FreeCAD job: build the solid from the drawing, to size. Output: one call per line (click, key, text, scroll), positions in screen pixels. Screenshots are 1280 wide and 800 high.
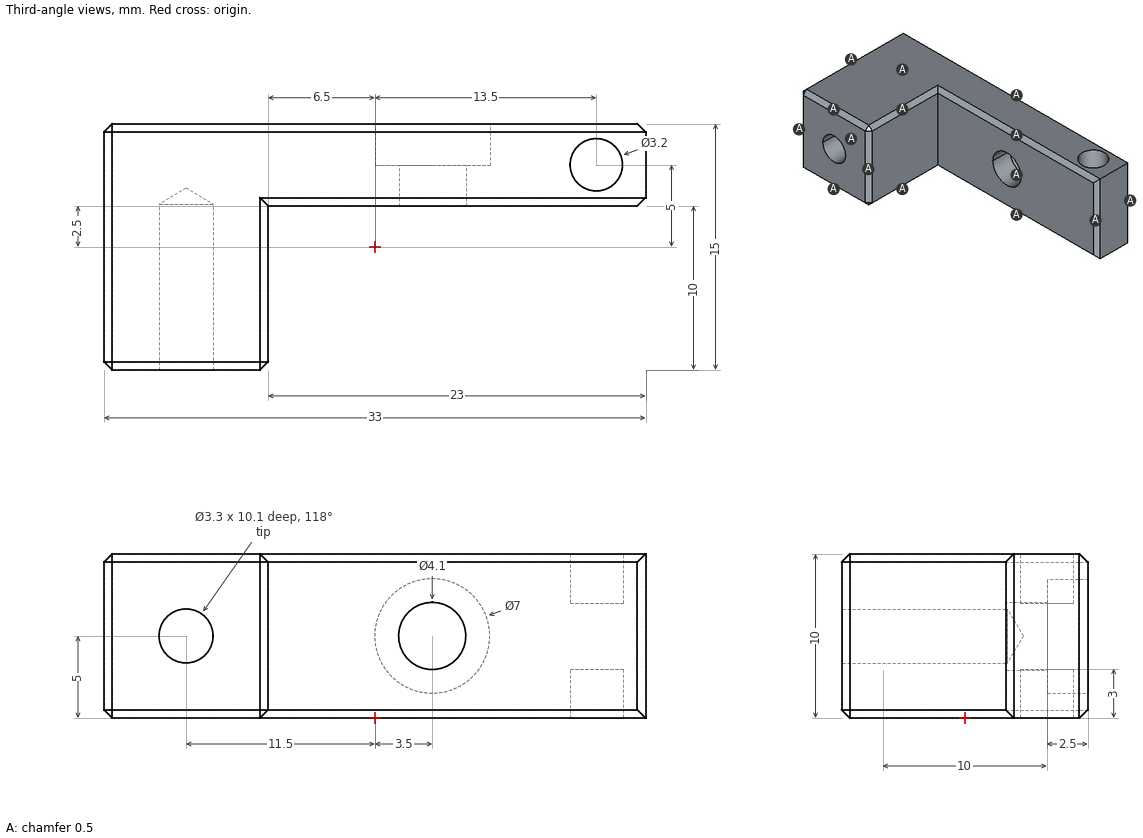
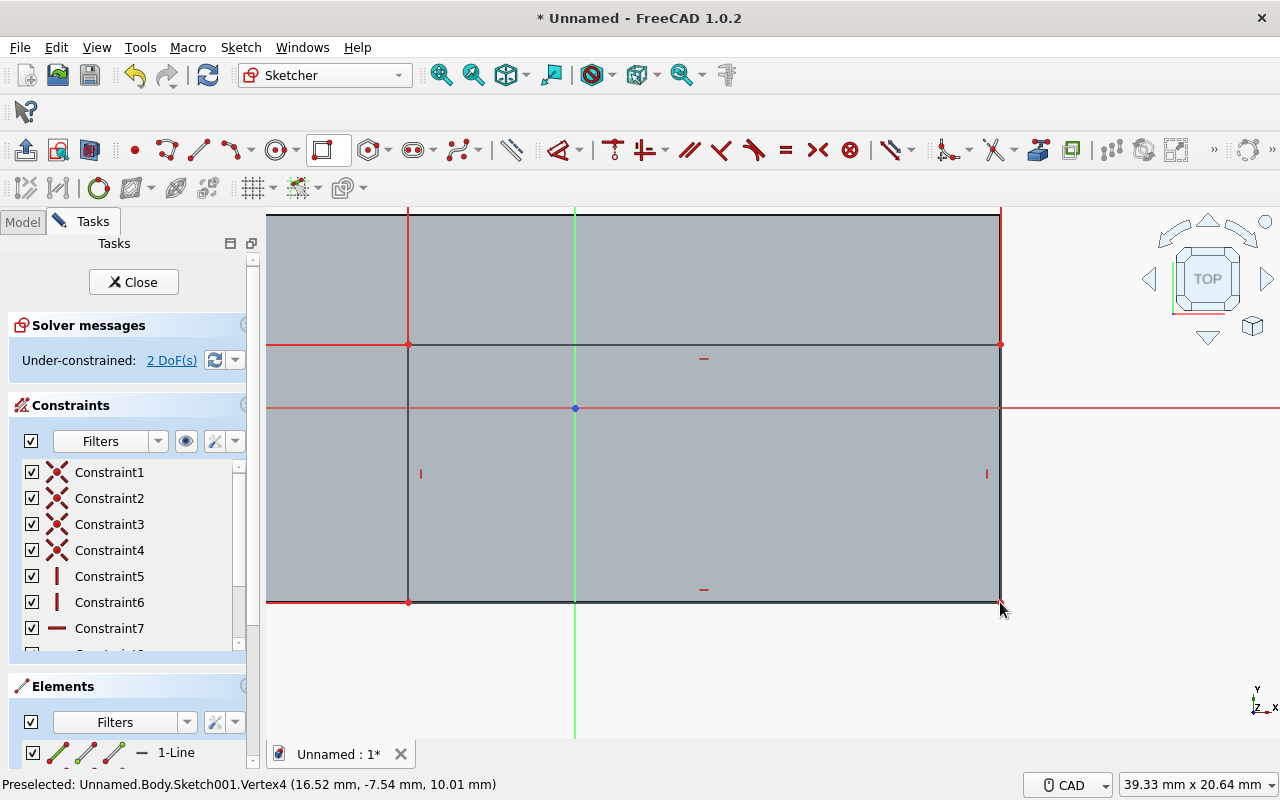
click(408, 345)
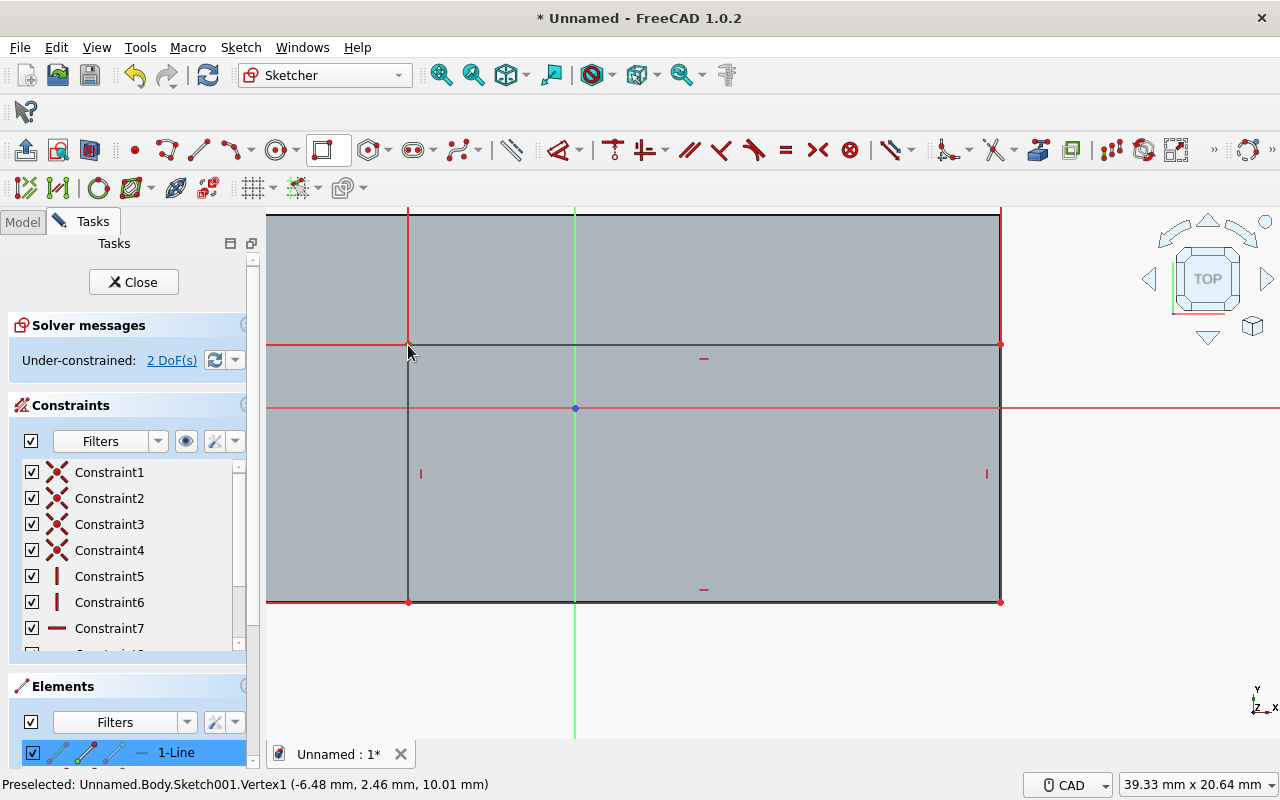
key(l)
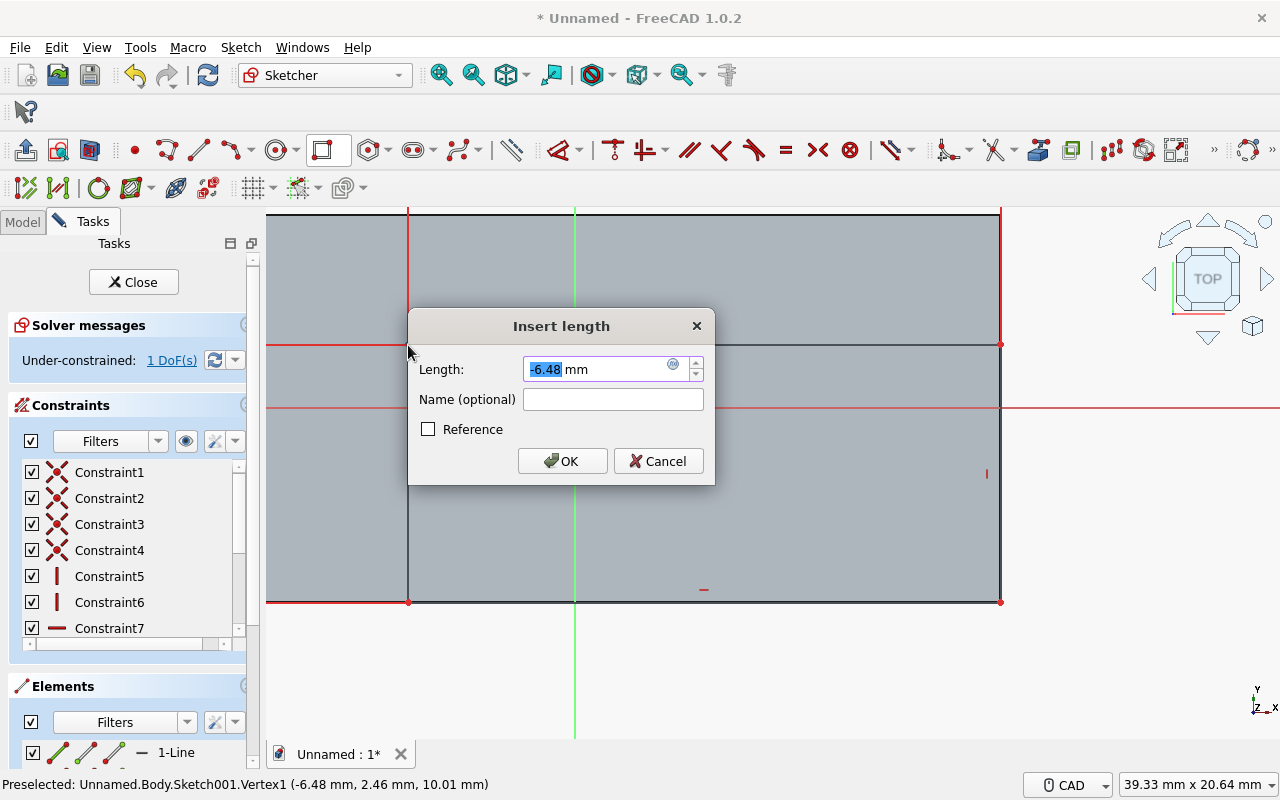
text(-6.5)
key(Return)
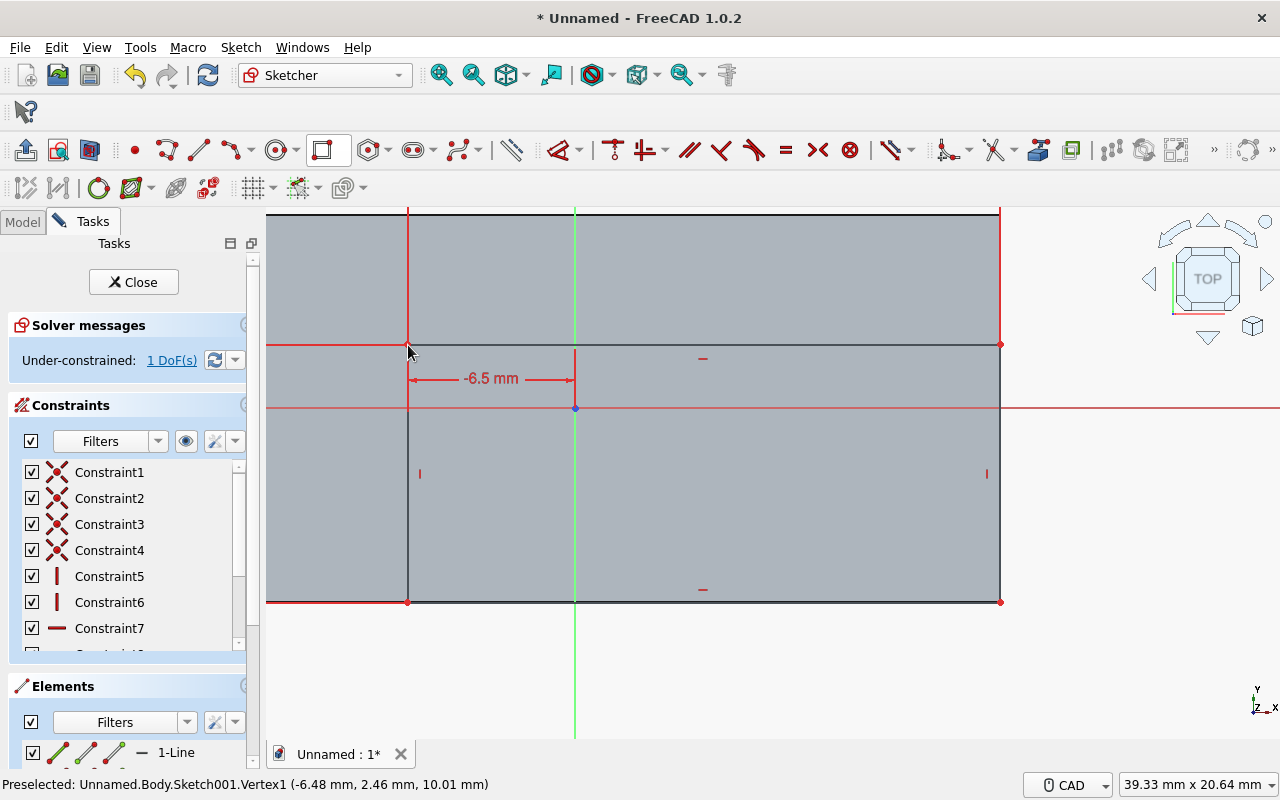
click(408, 345)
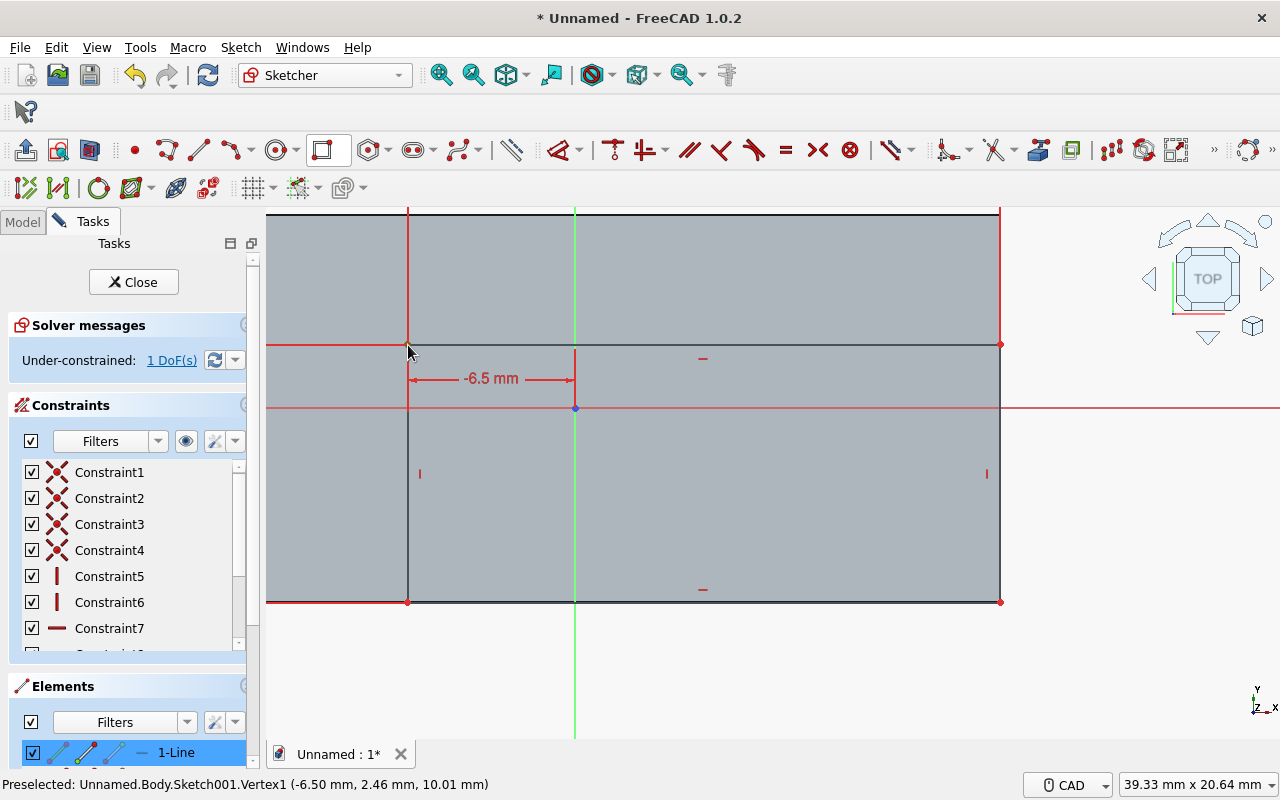
key(i)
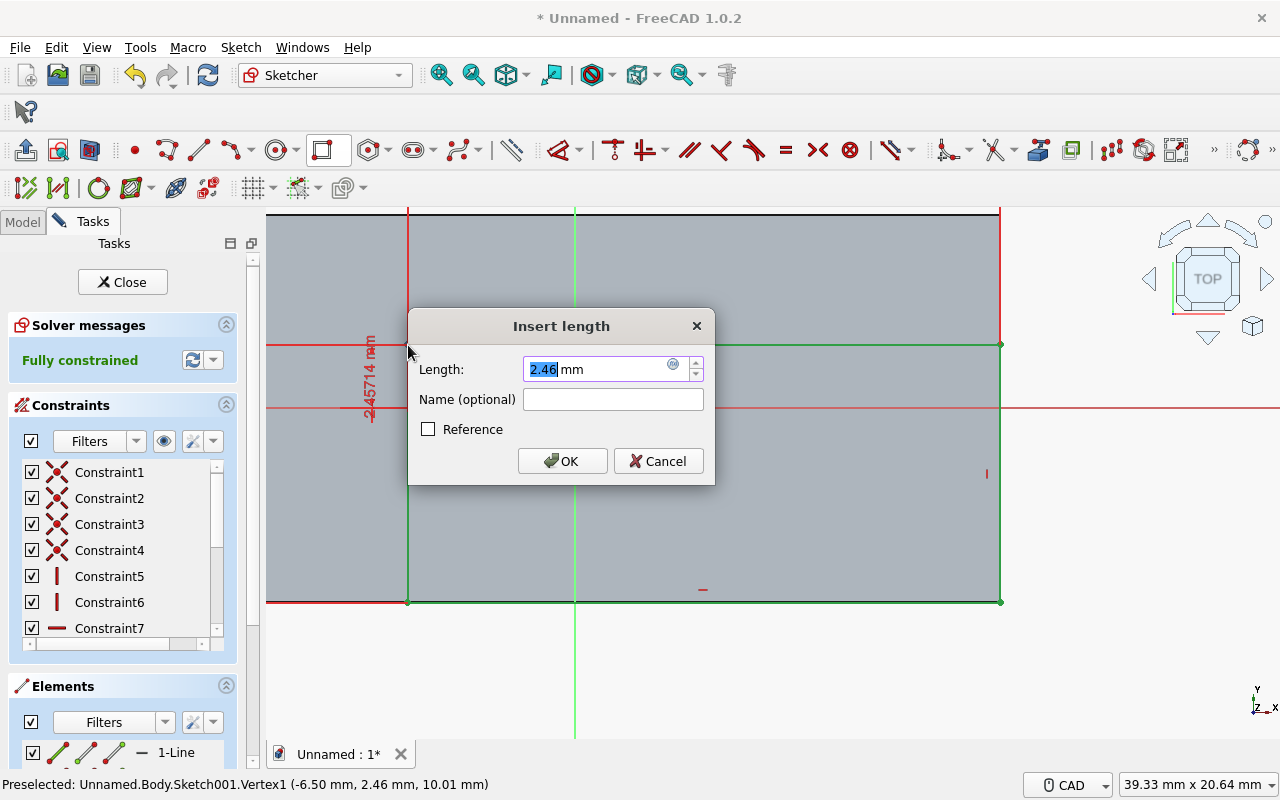
text(2.5)
key(Return)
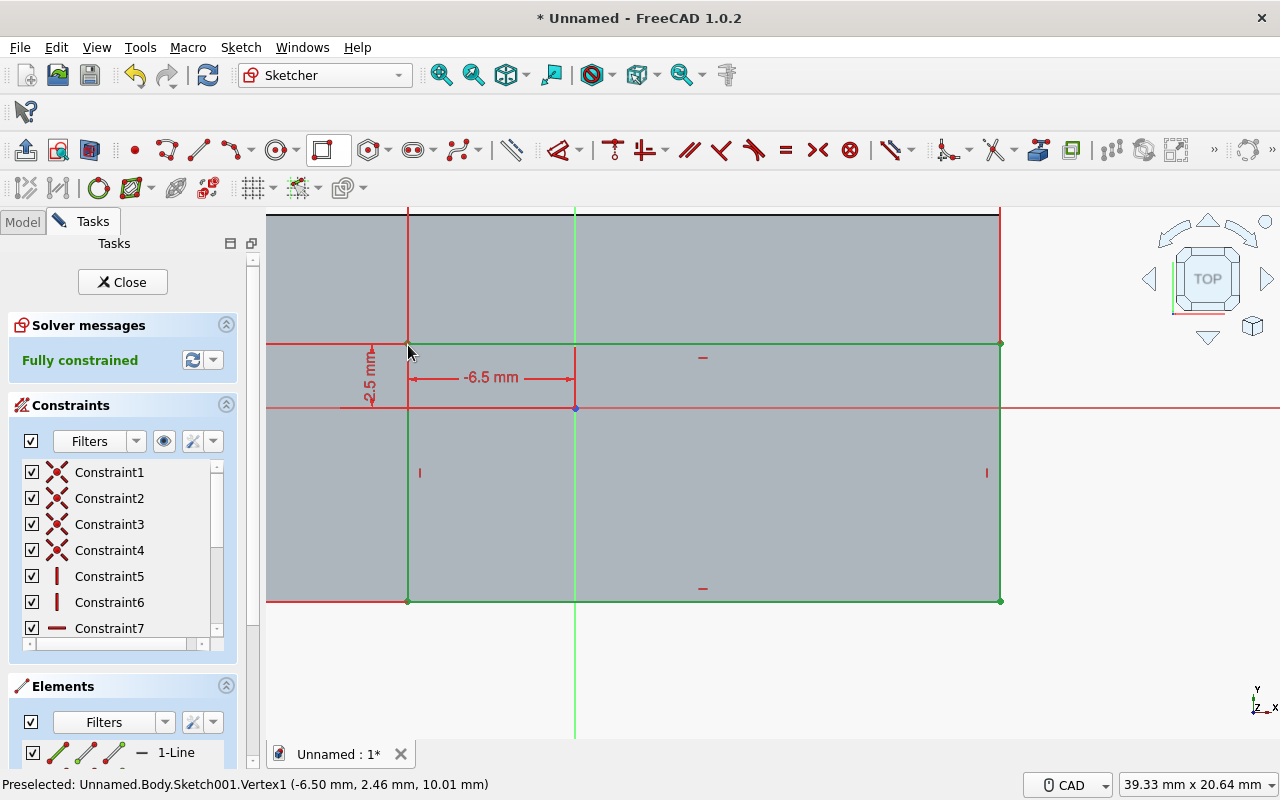
click(123, 282)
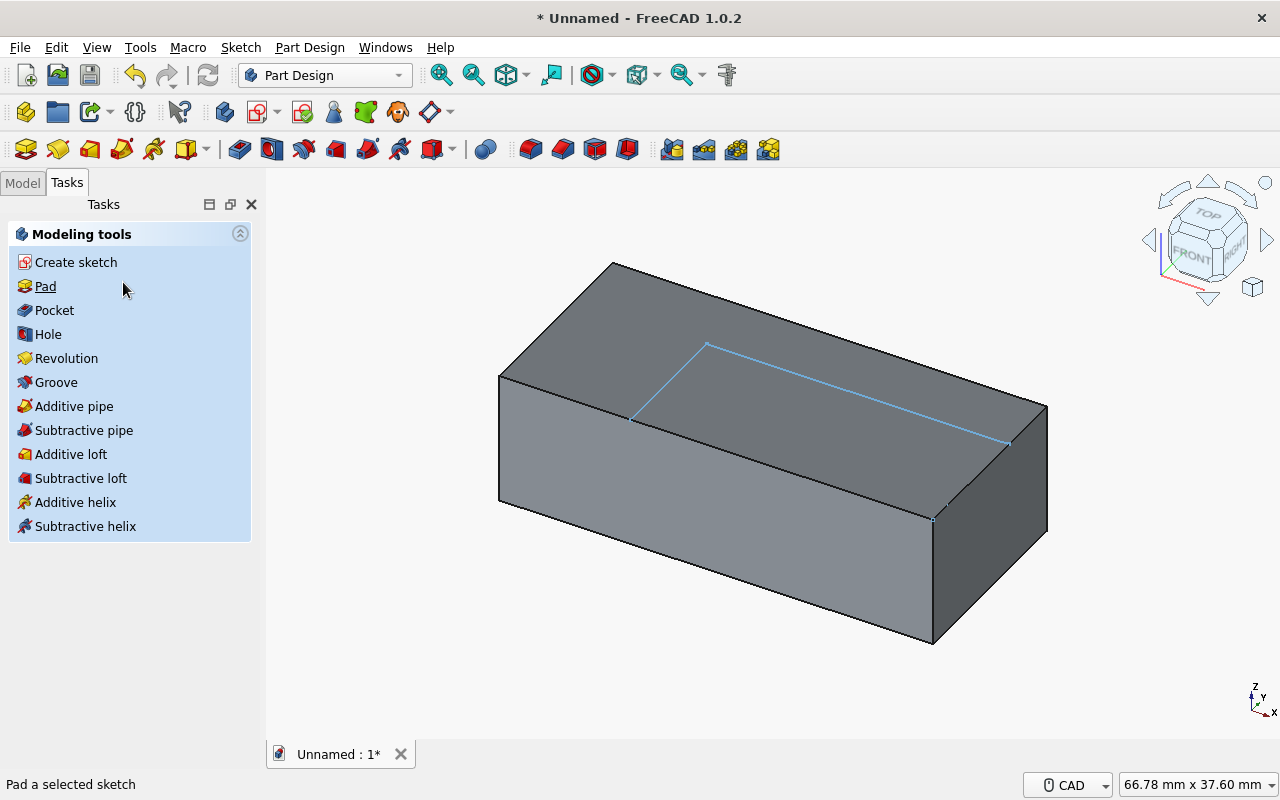
click(240, 150)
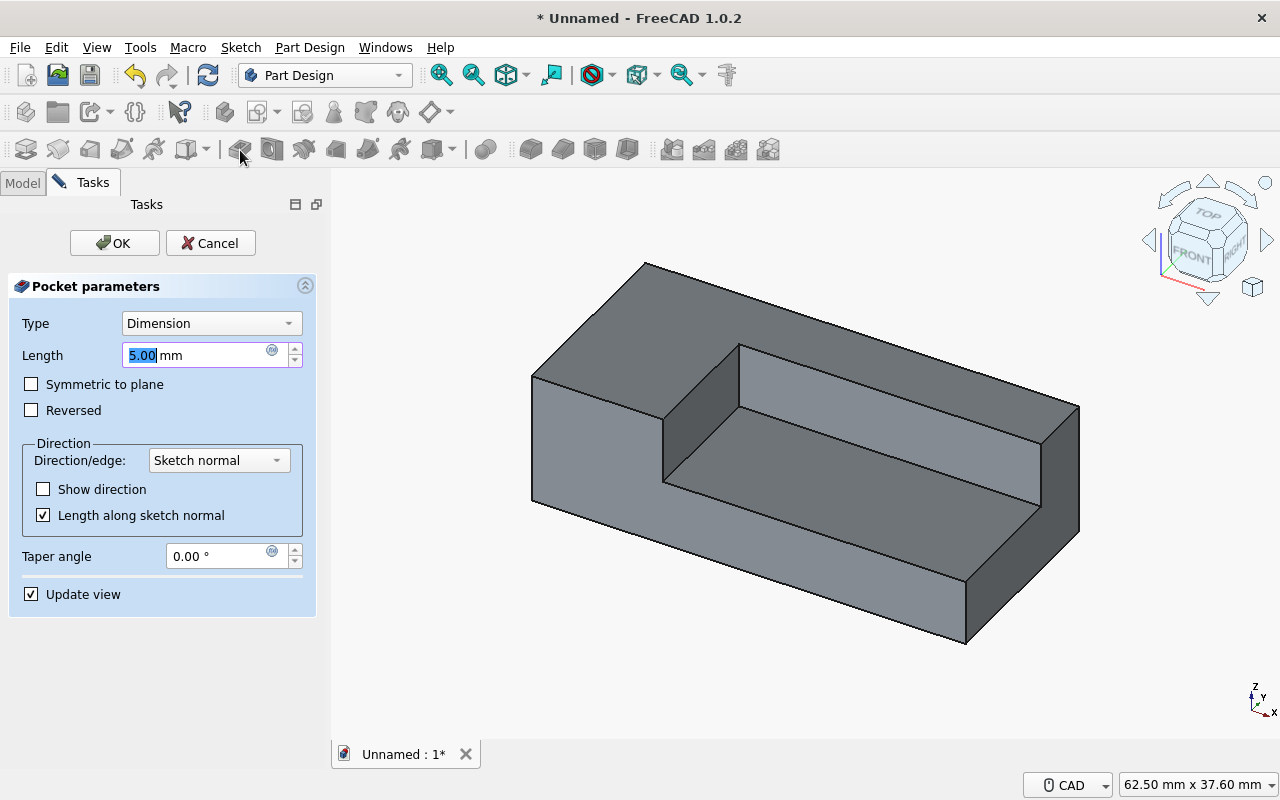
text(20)
key(Tab)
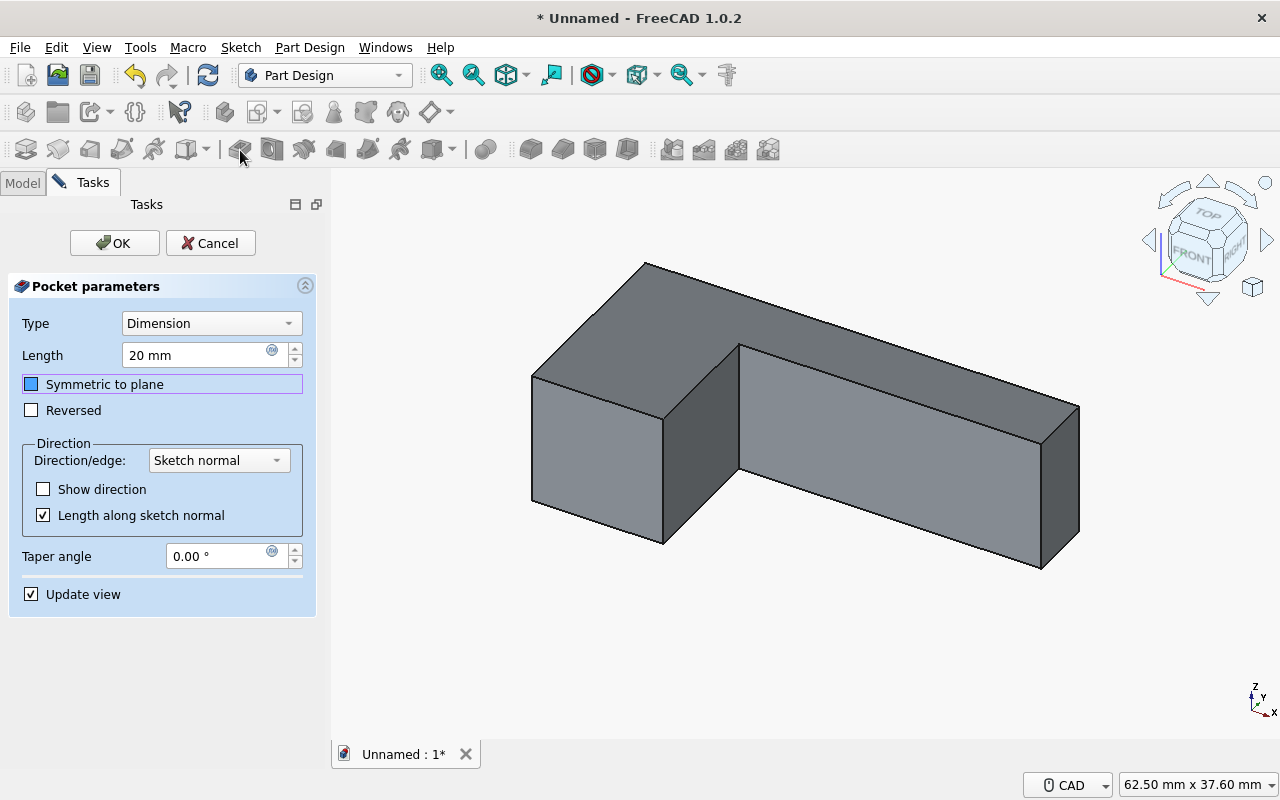
click(115, 243)